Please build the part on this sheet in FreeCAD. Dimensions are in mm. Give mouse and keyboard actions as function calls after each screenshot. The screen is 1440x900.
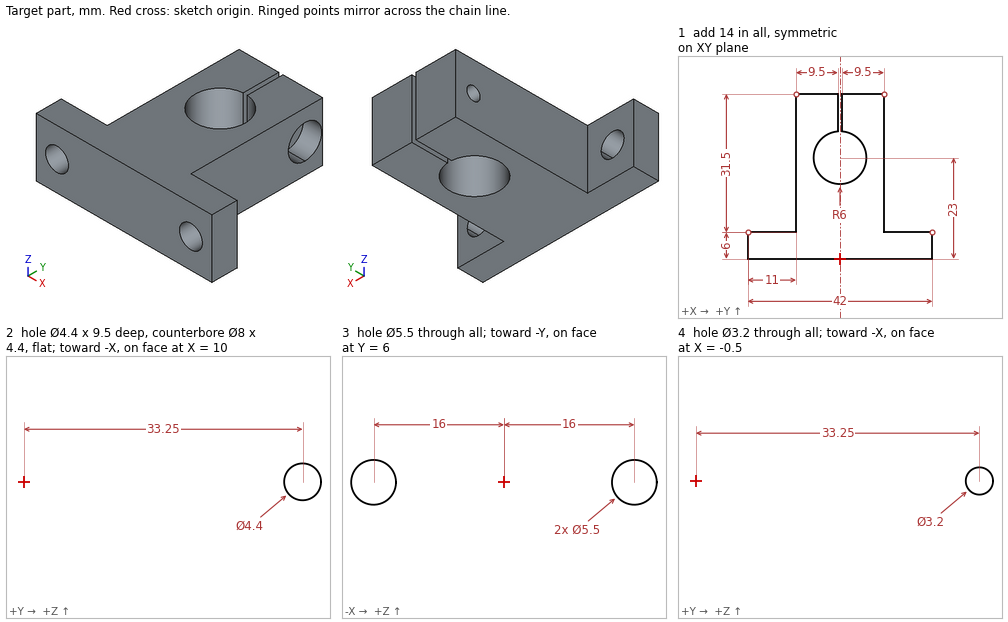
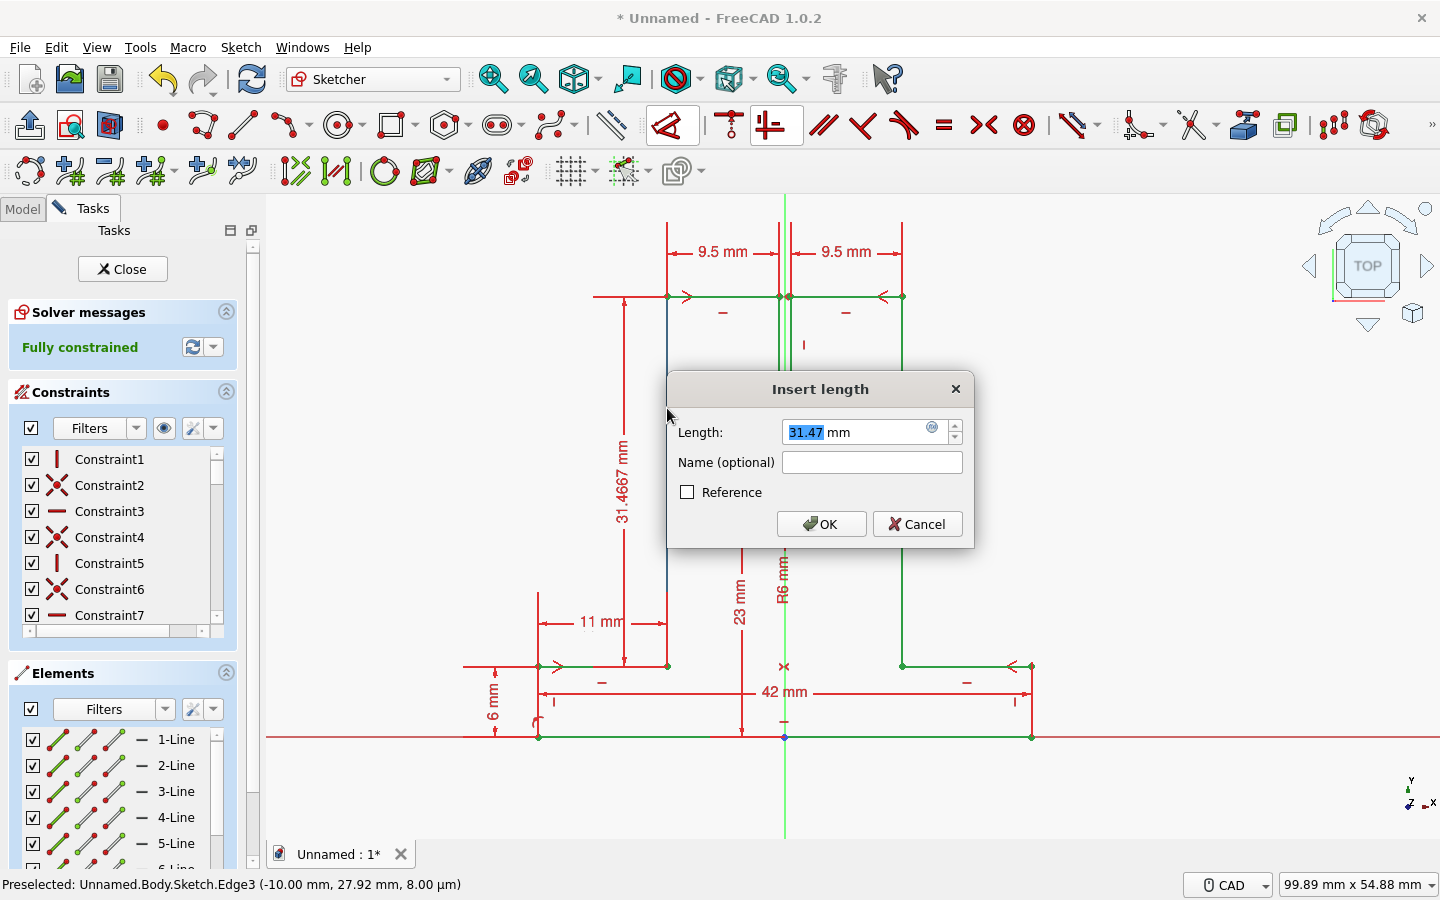
text(31.5)
key(Return)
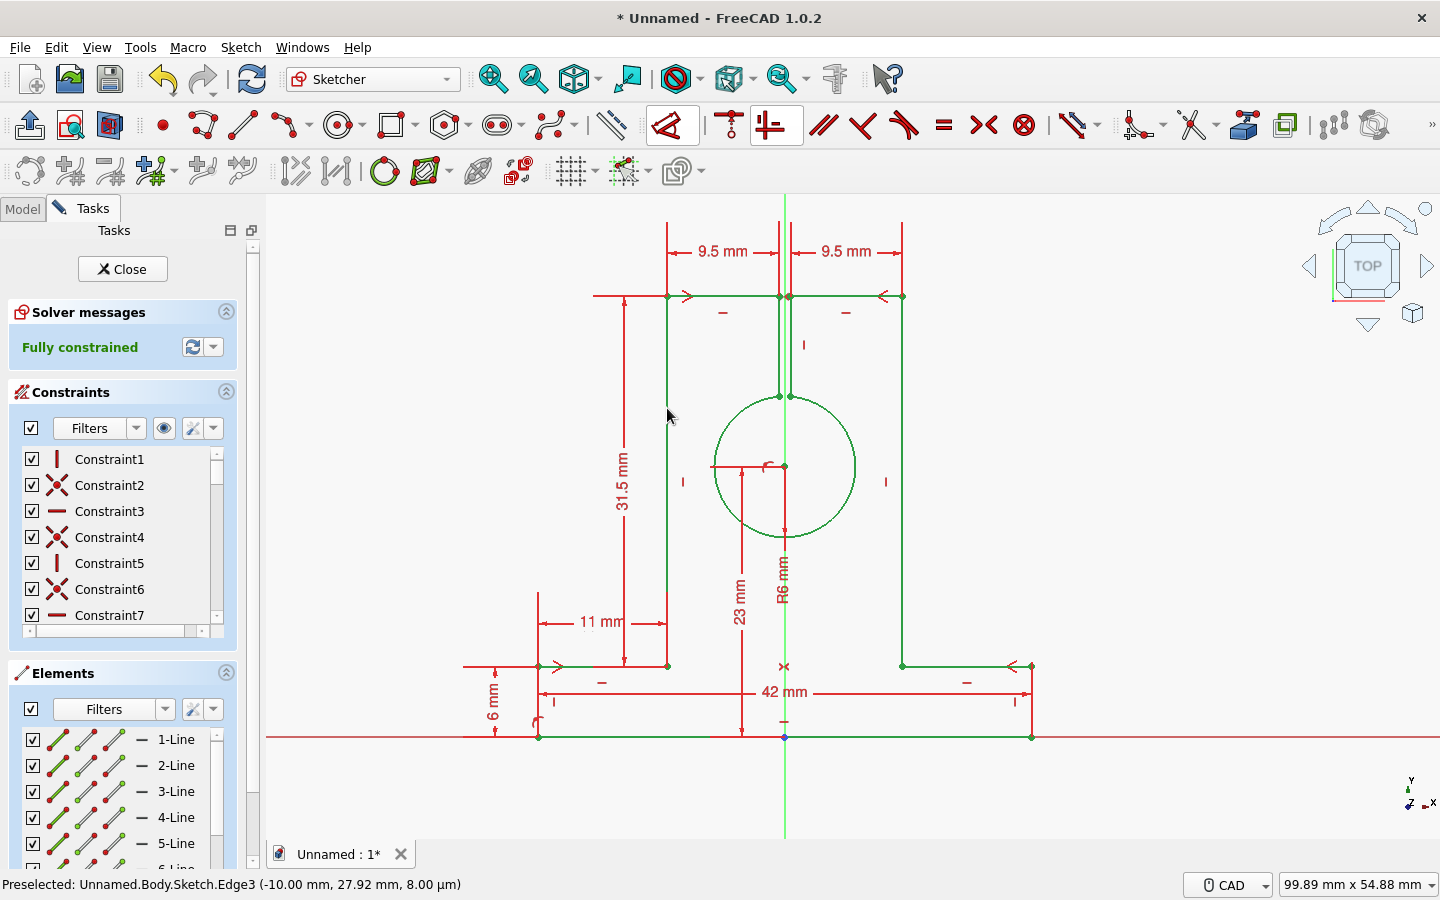
click(123, 269)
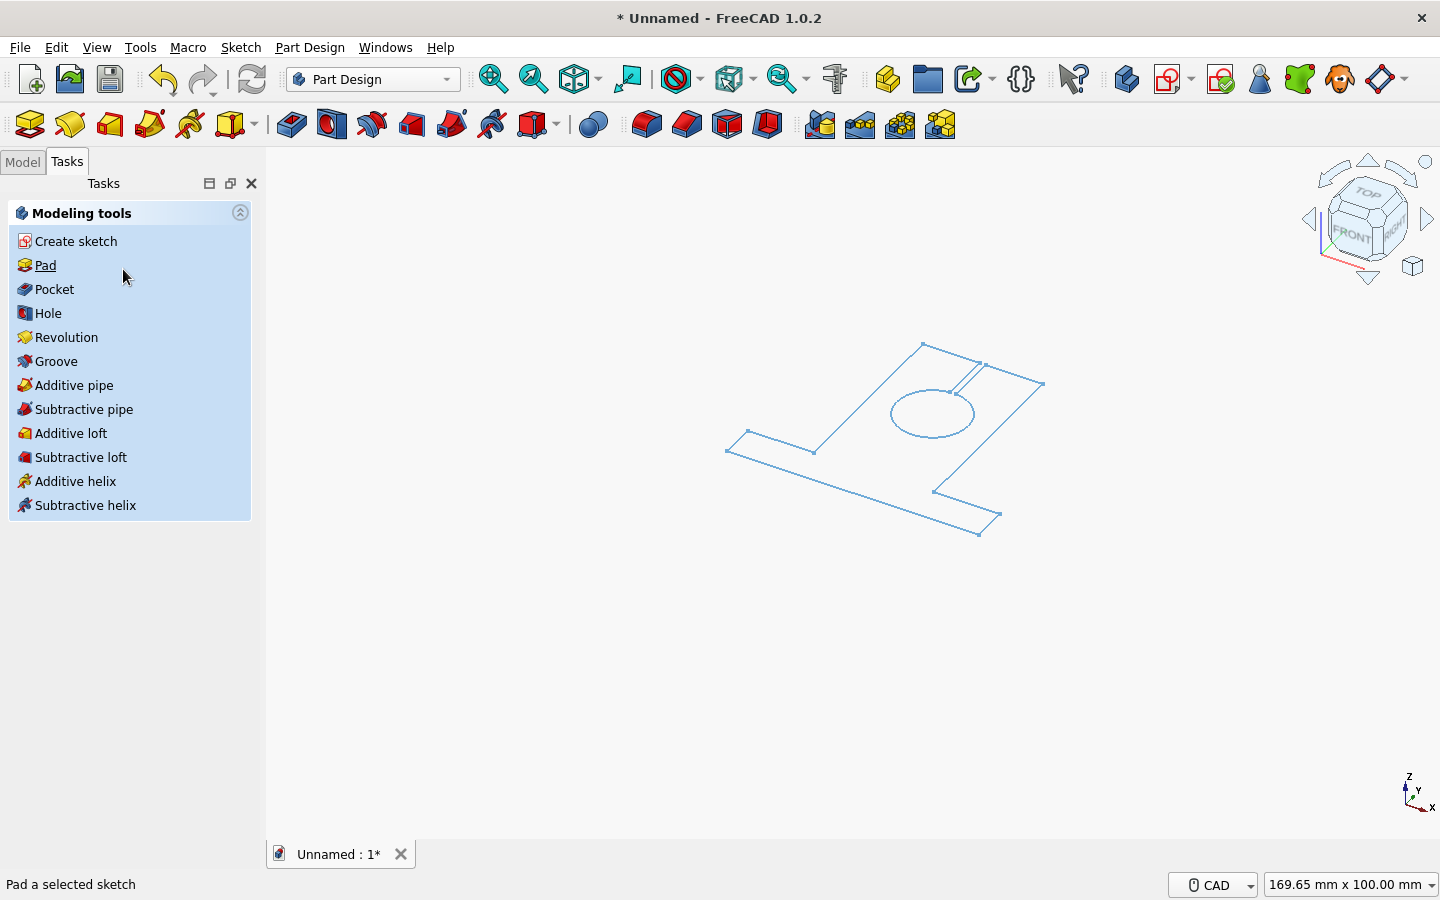
click(30, 124)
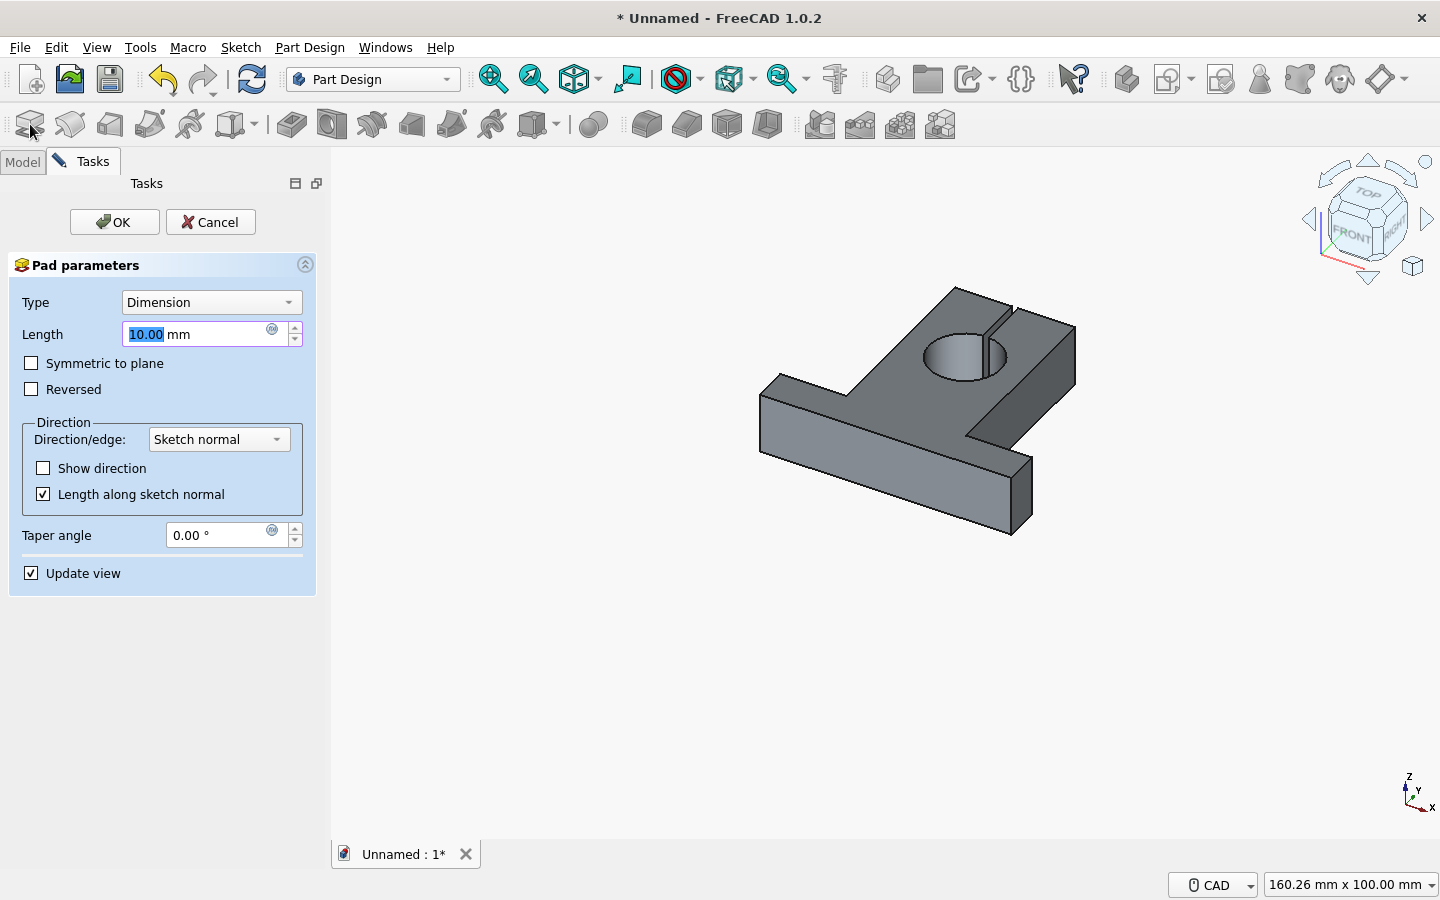
text(14)
key(Tab)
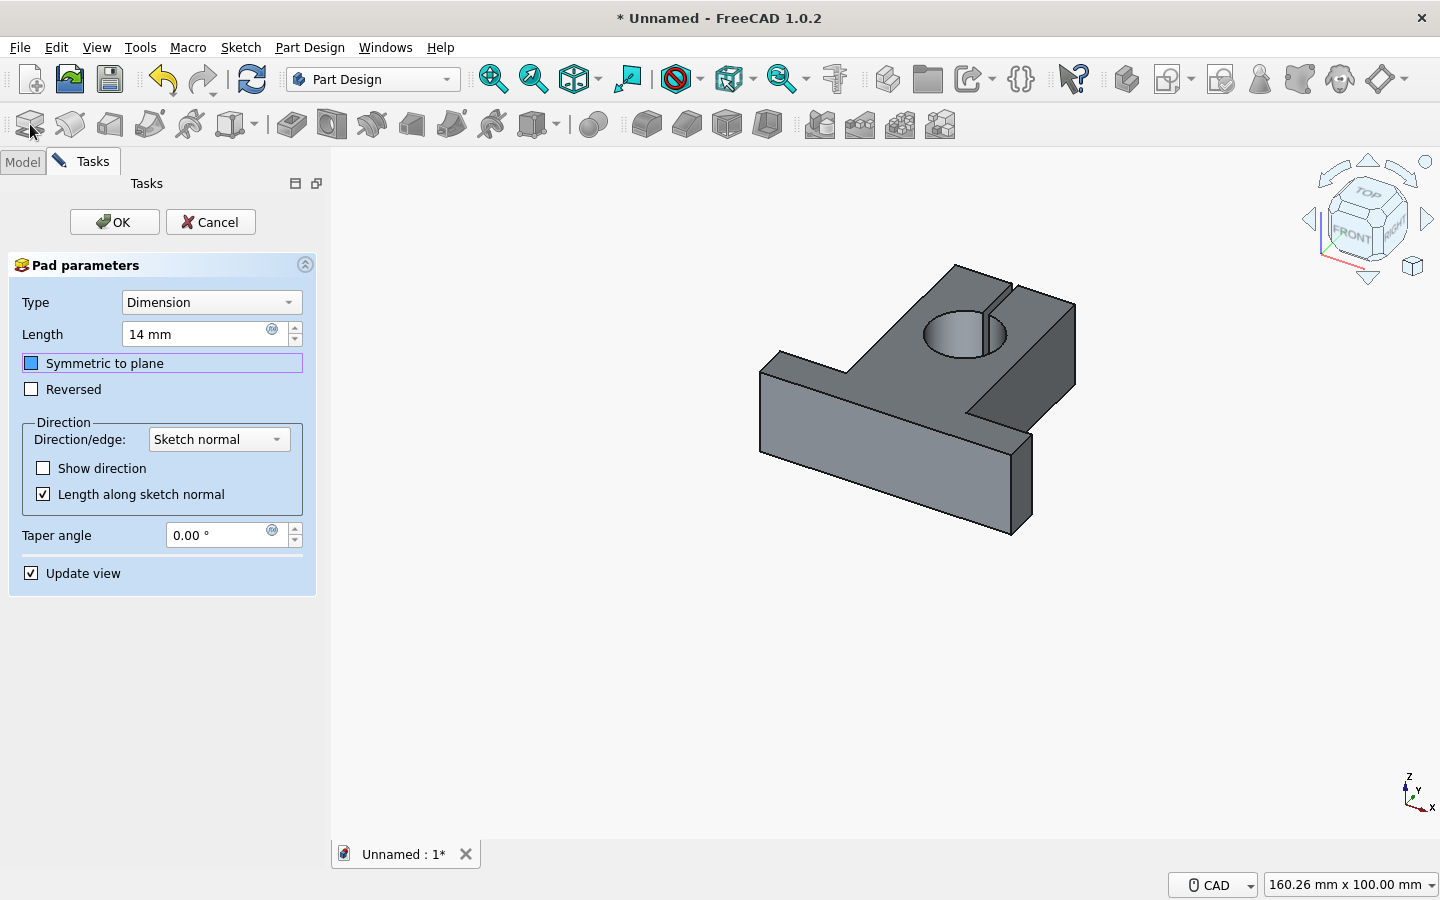
click(30, 363)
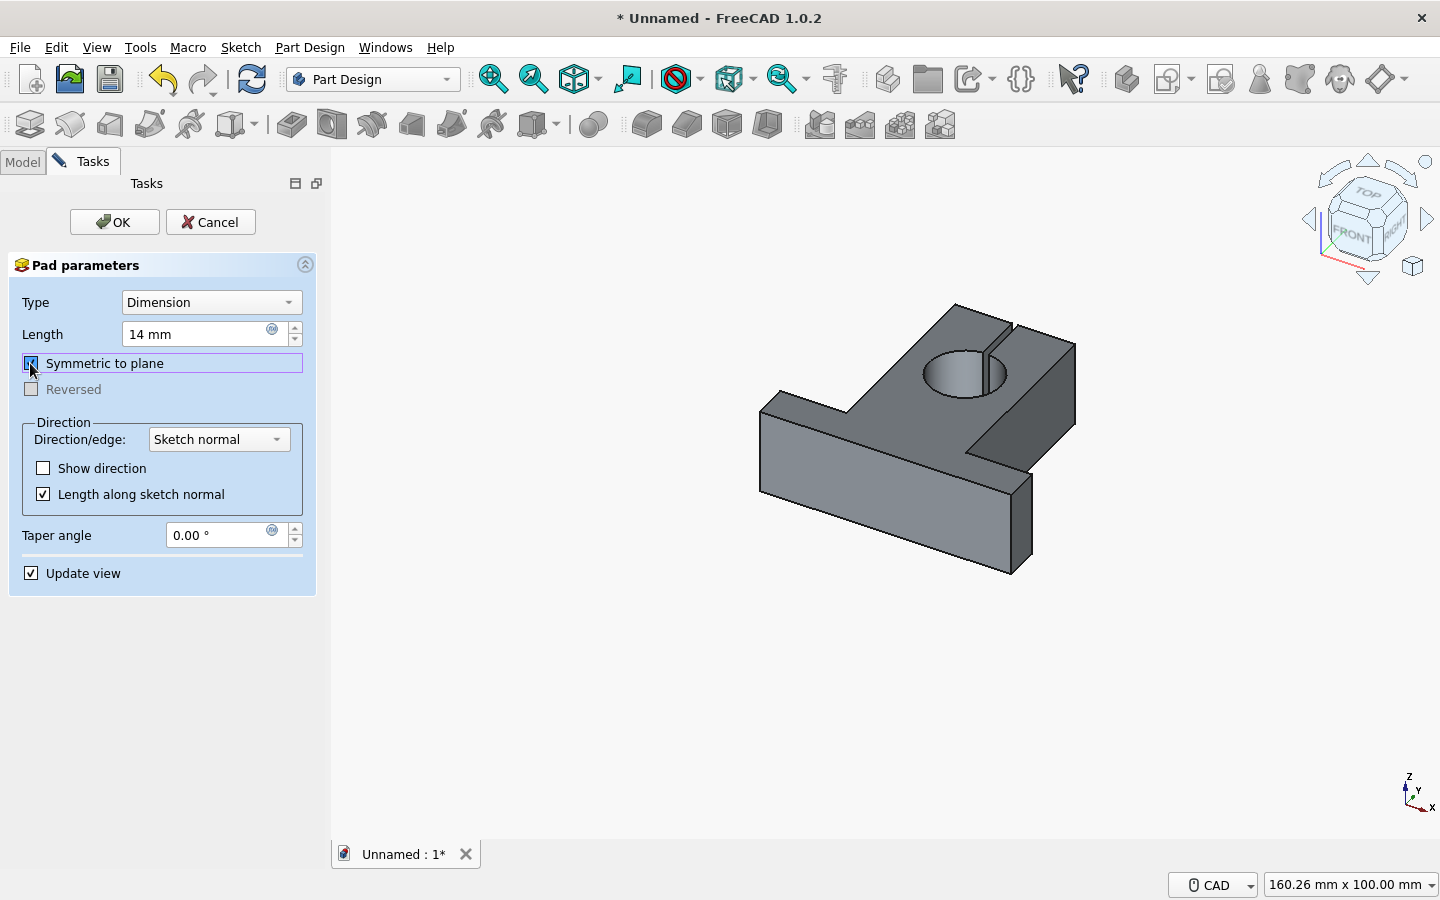
click(115, 222)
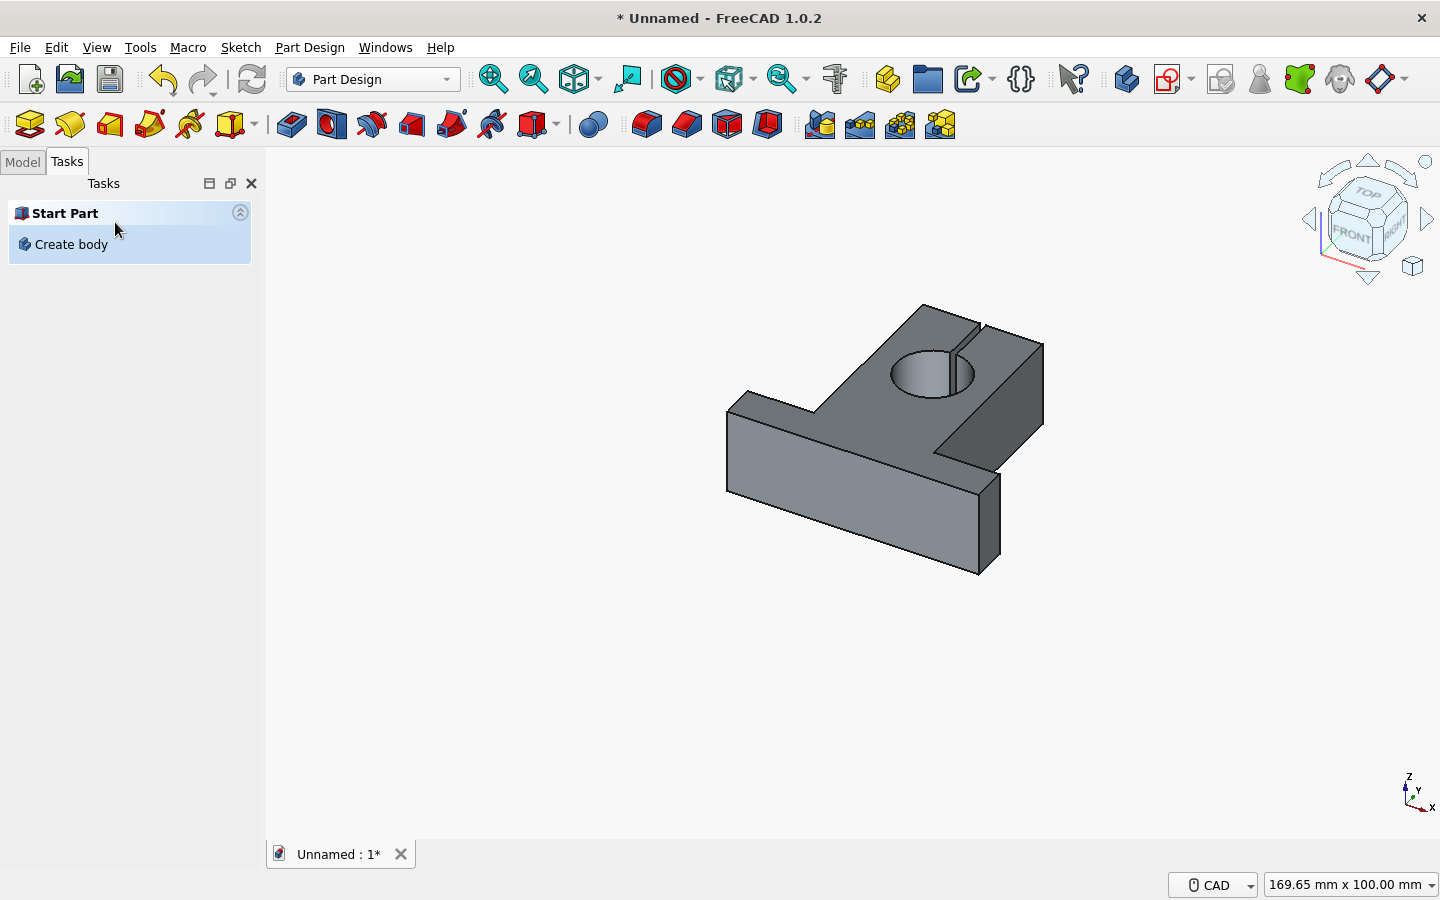
click(494, 80)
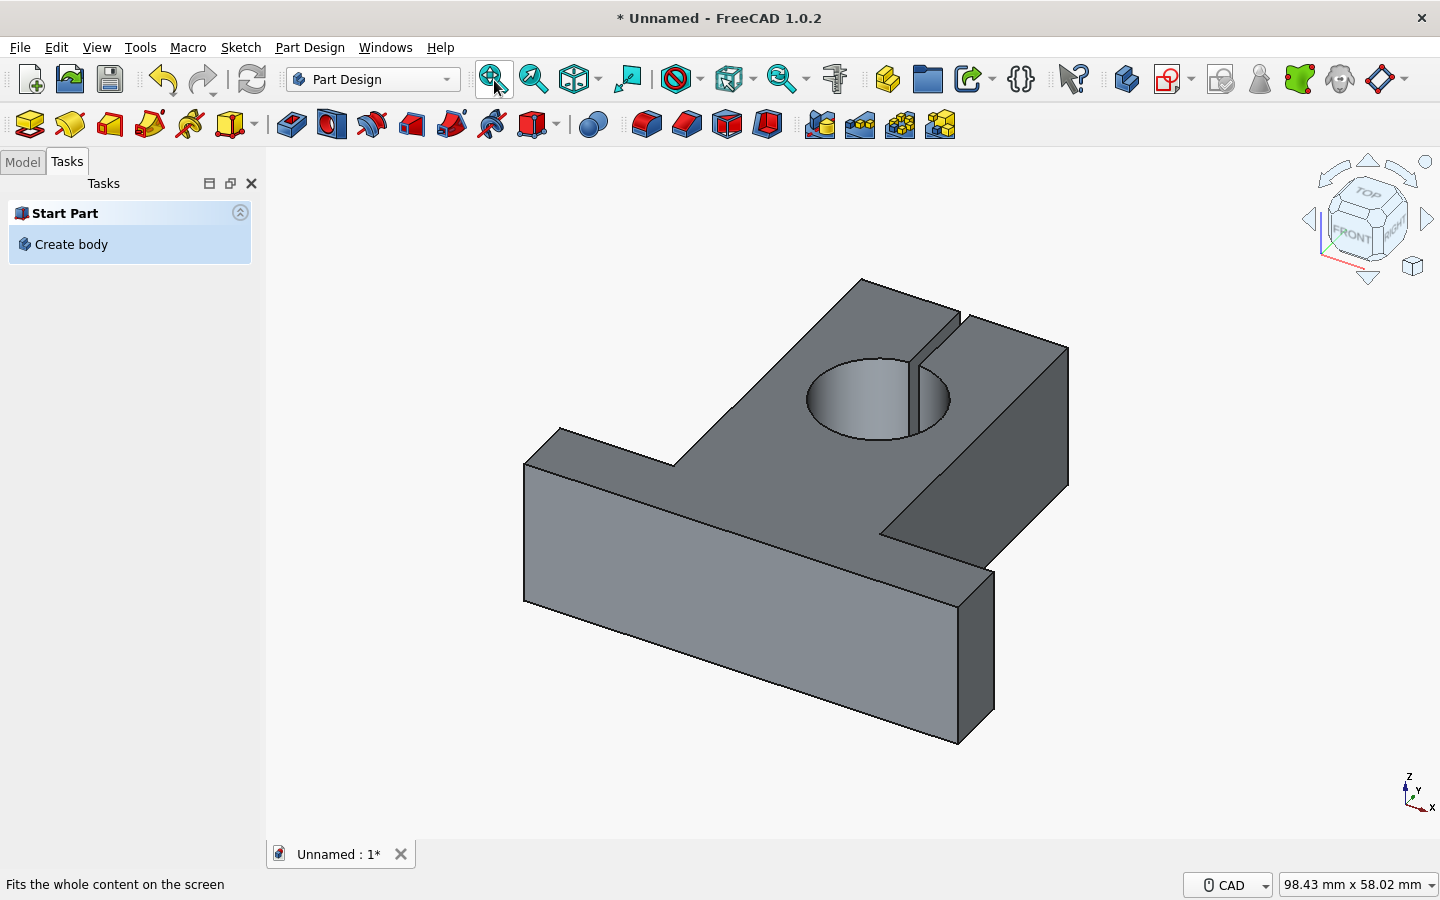
click(1001, 482)